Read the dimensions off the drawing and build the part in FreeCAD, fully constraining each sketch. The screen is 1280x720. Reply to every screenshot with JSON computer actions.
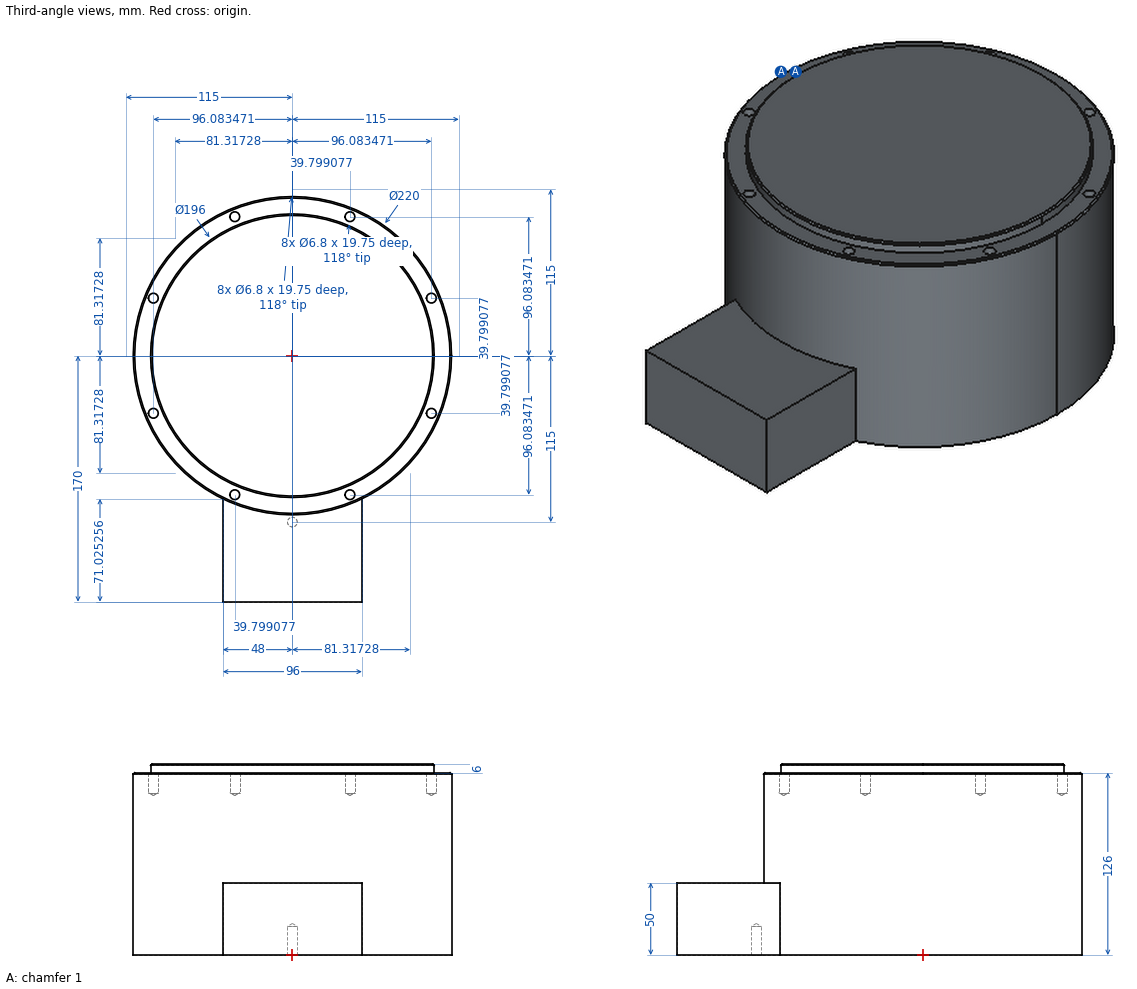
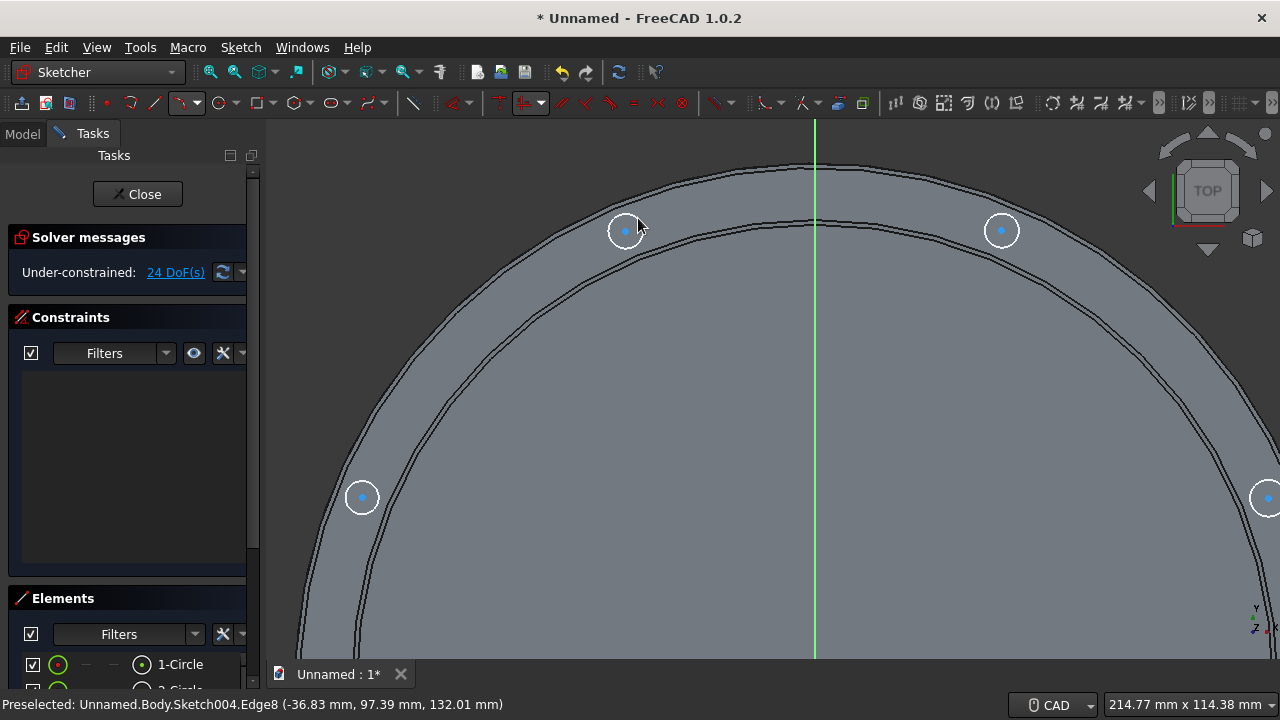
{"action": "left_click", "coordinate": [1014, 219]}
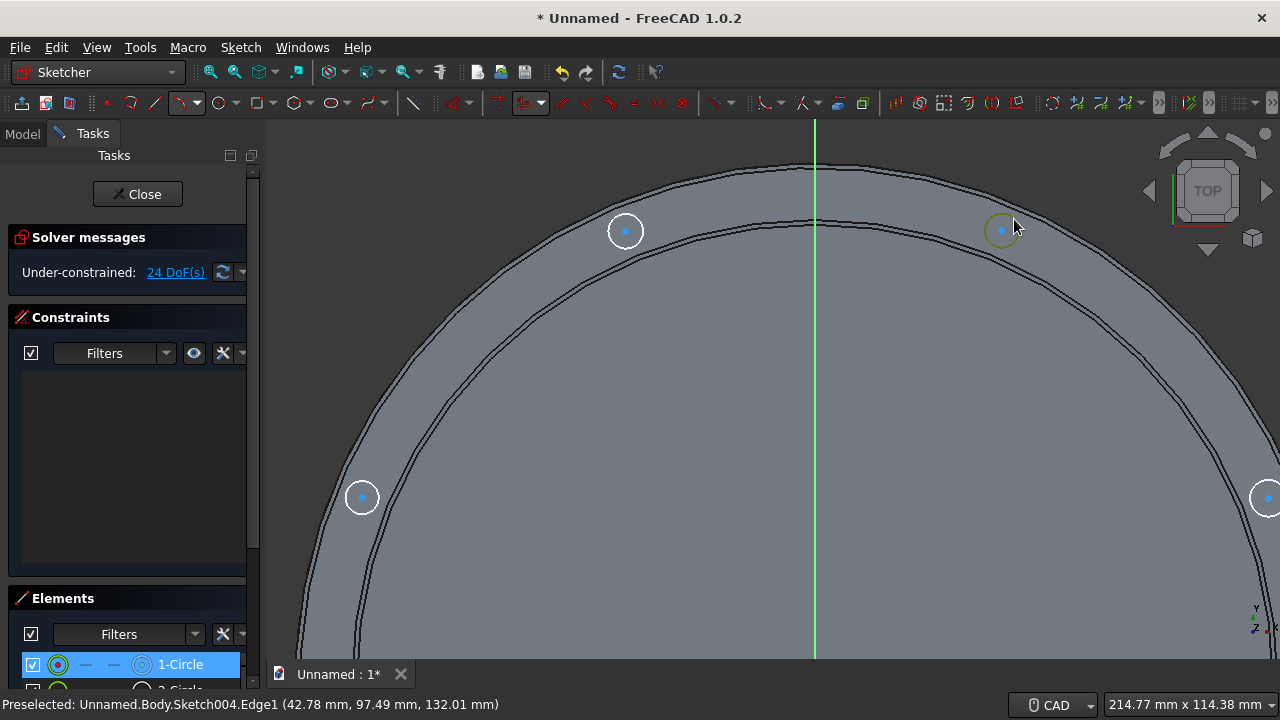
{"action": "scroll", "coordinate": [640, 218], "scroll_direction": "down", "scroll_amount": 5}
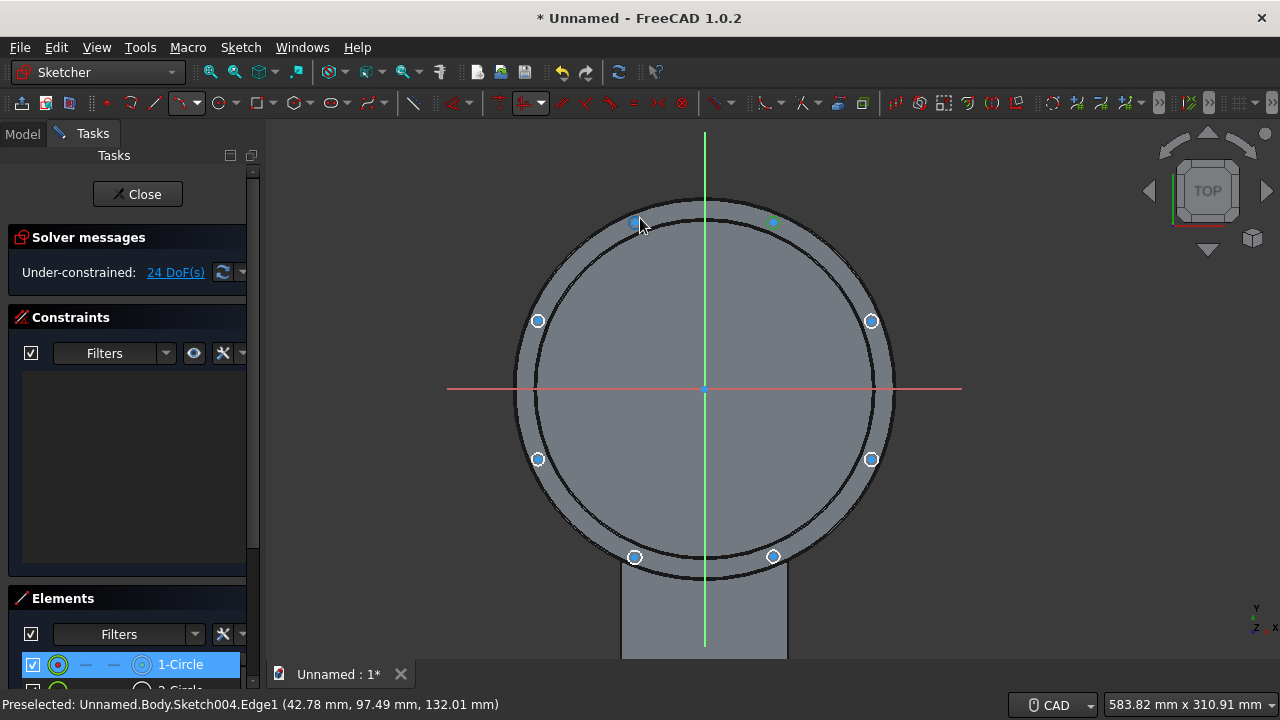
{"action": "scroll", "coordinate": [876, 316], "scroll_direction": "up", "scroll_amount": 4}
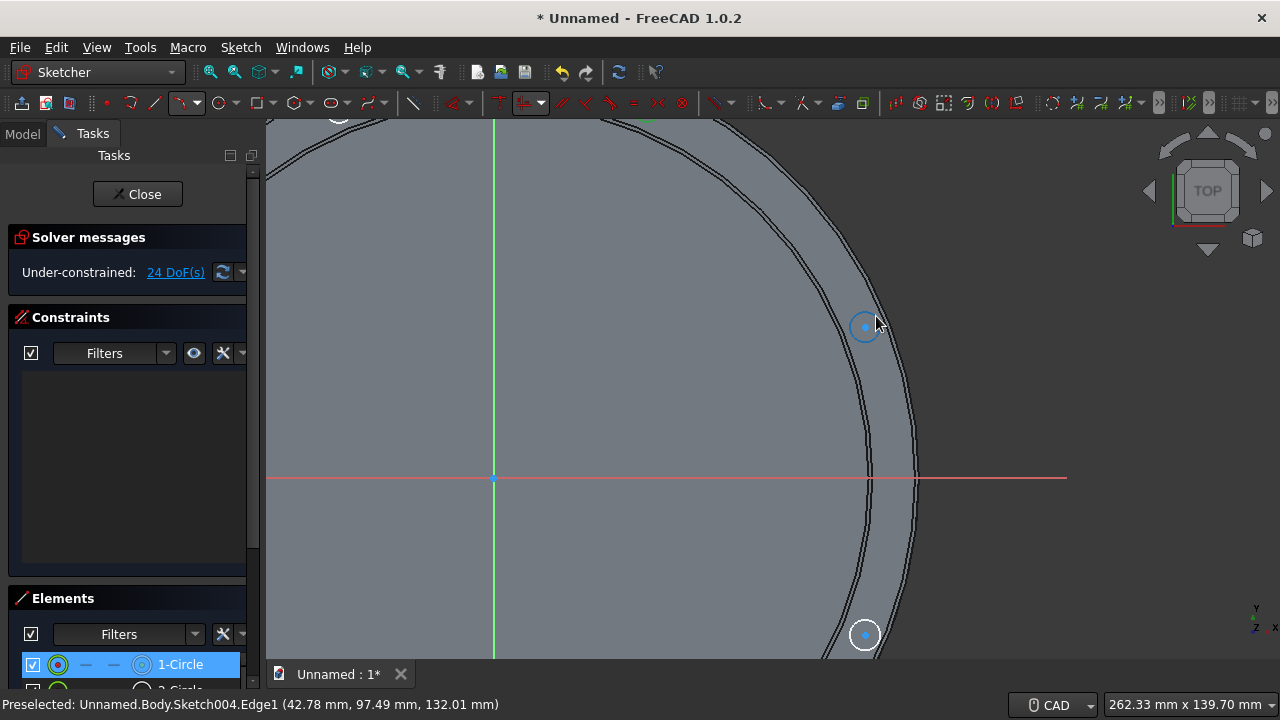
{"action": "left_click", "coordinate": [876, 316]}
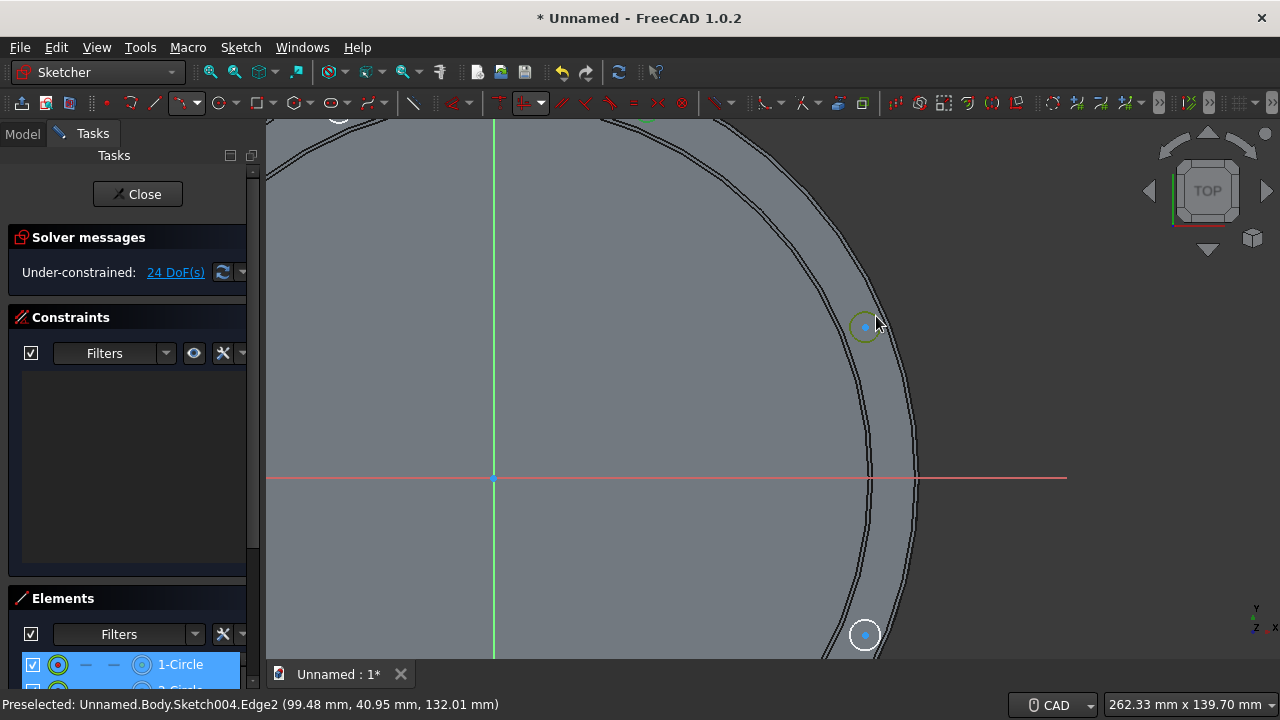
{"action": "left_click", "coordinate": [876, 624]}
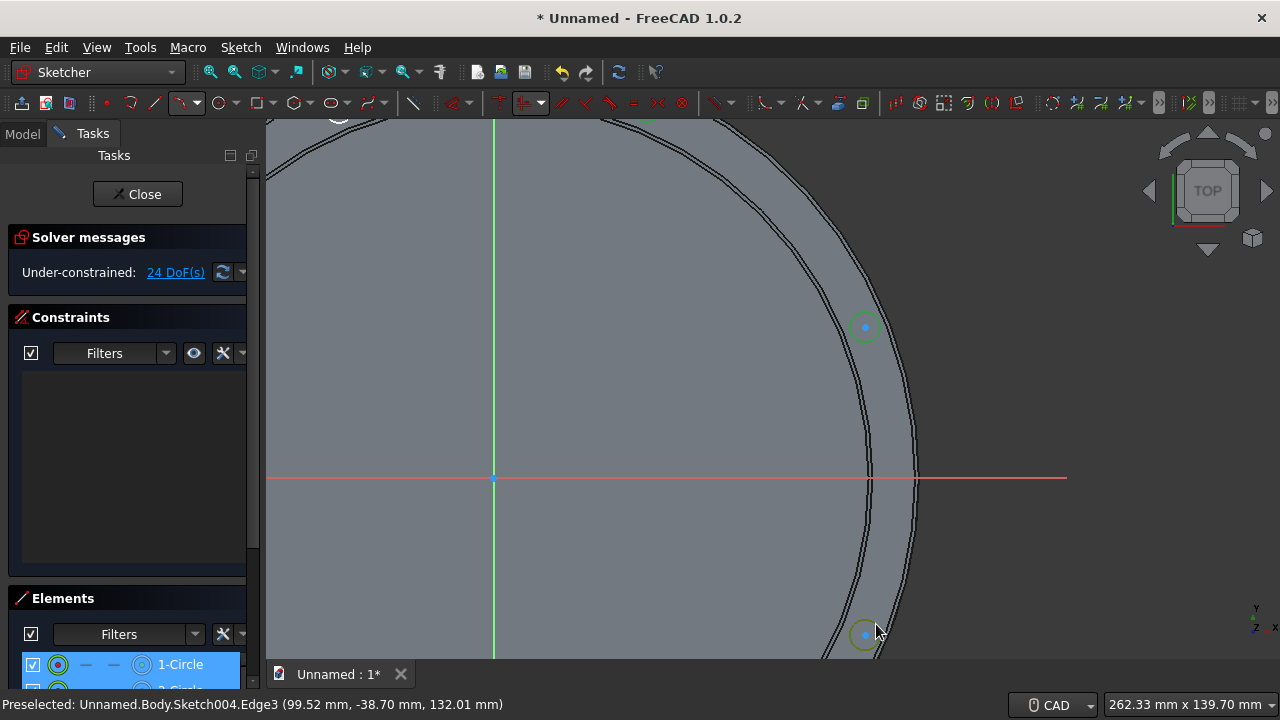
{"action": "scroll", "coordinate": [877, 316], "scroll_direction": "down", "scroll_amount": 4}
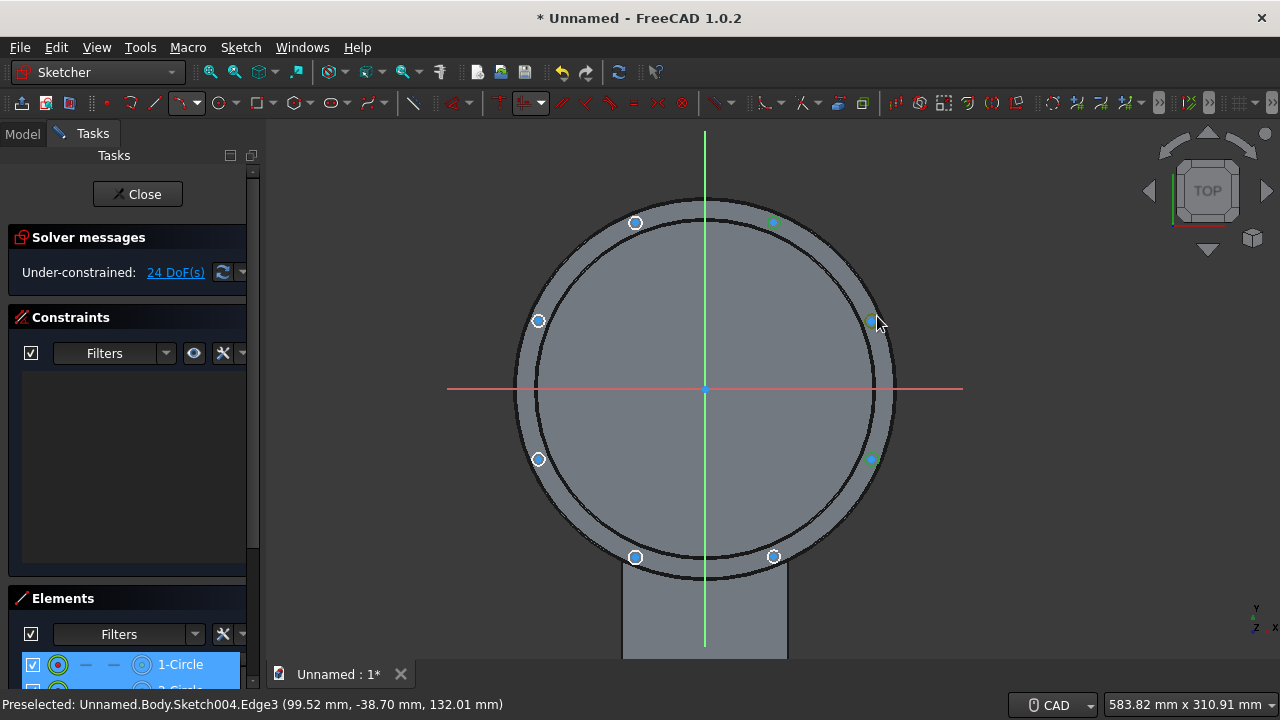
{"action": "scroll", "coordinate": [778, 552], "scroll_direction": "up", "scroll_amount": 4}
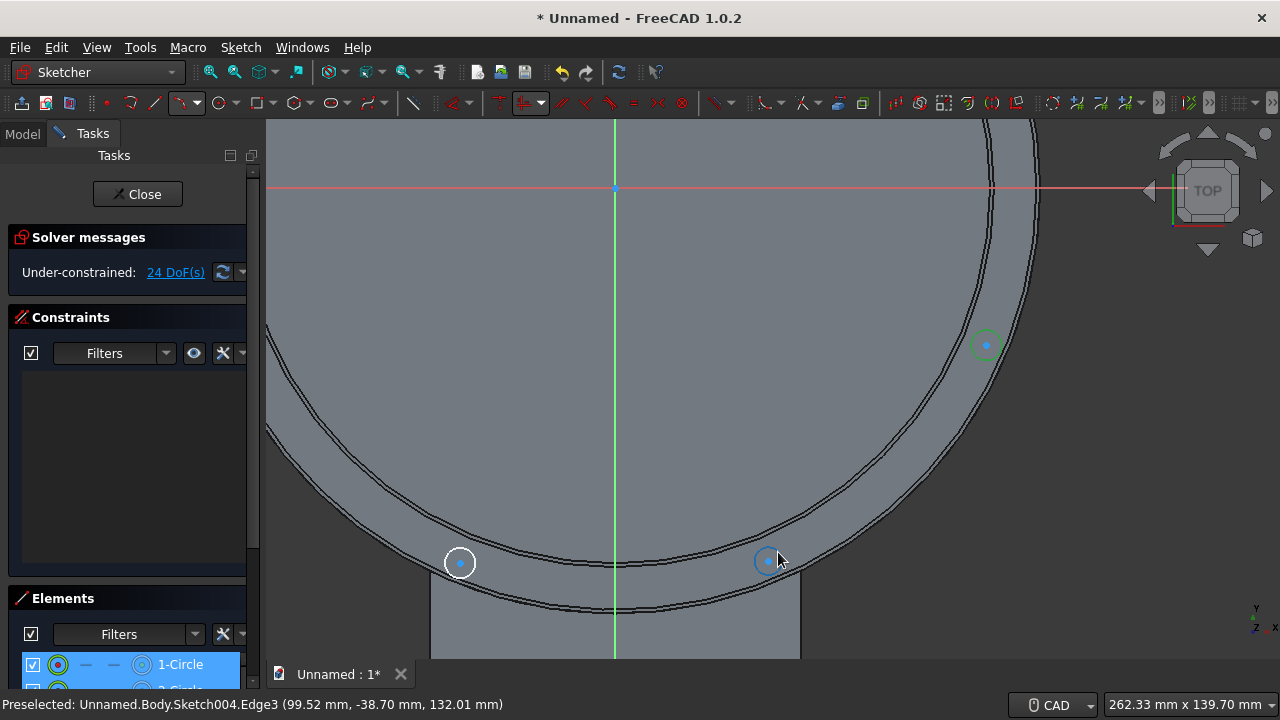
{"action": "left_click", "coordinate": [778, 551]}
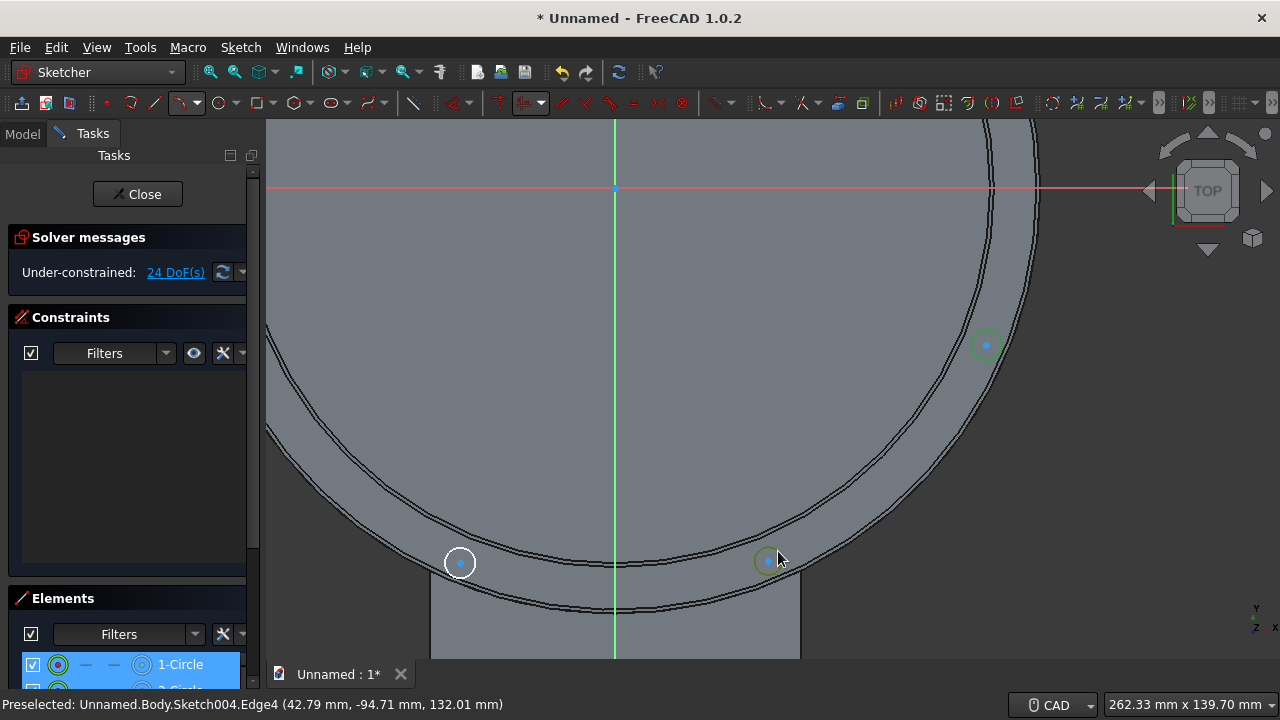
{"action": "left_click", "coordinate": [471, 552]}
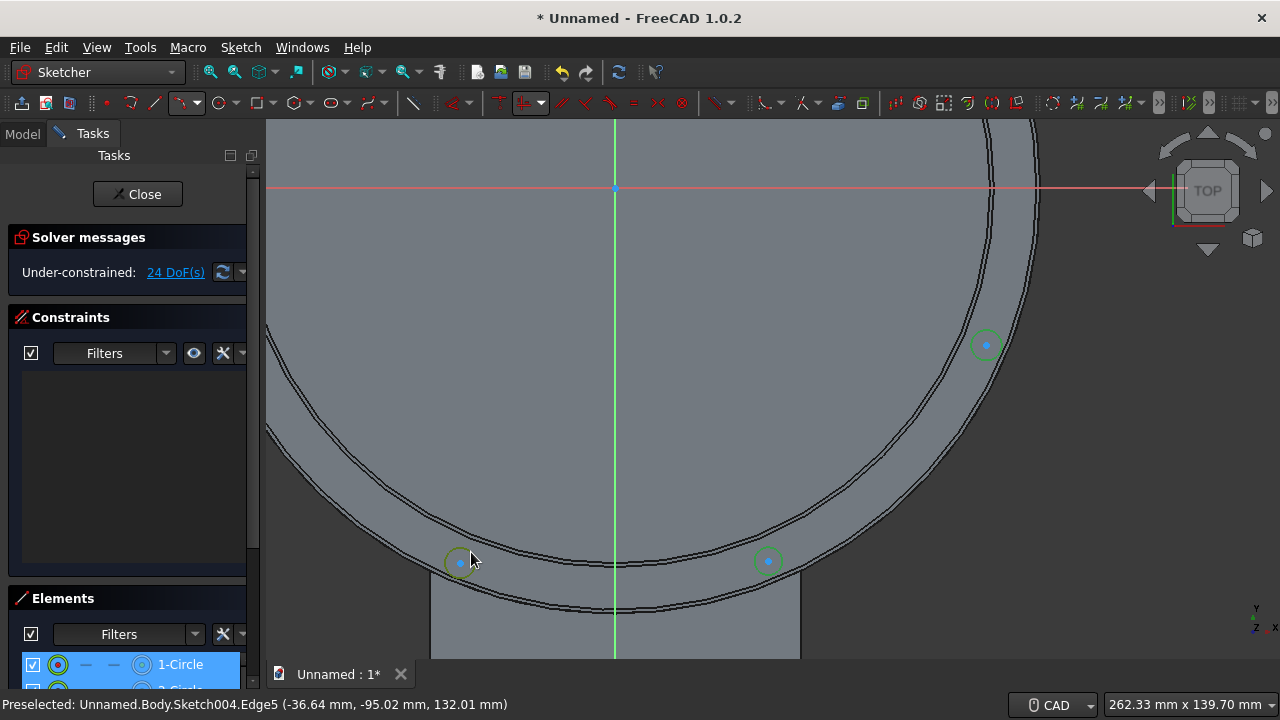
{"action": "scroll", "coordinate": [777, 553], "scroll_direction": "down", "scroll_amount": 4}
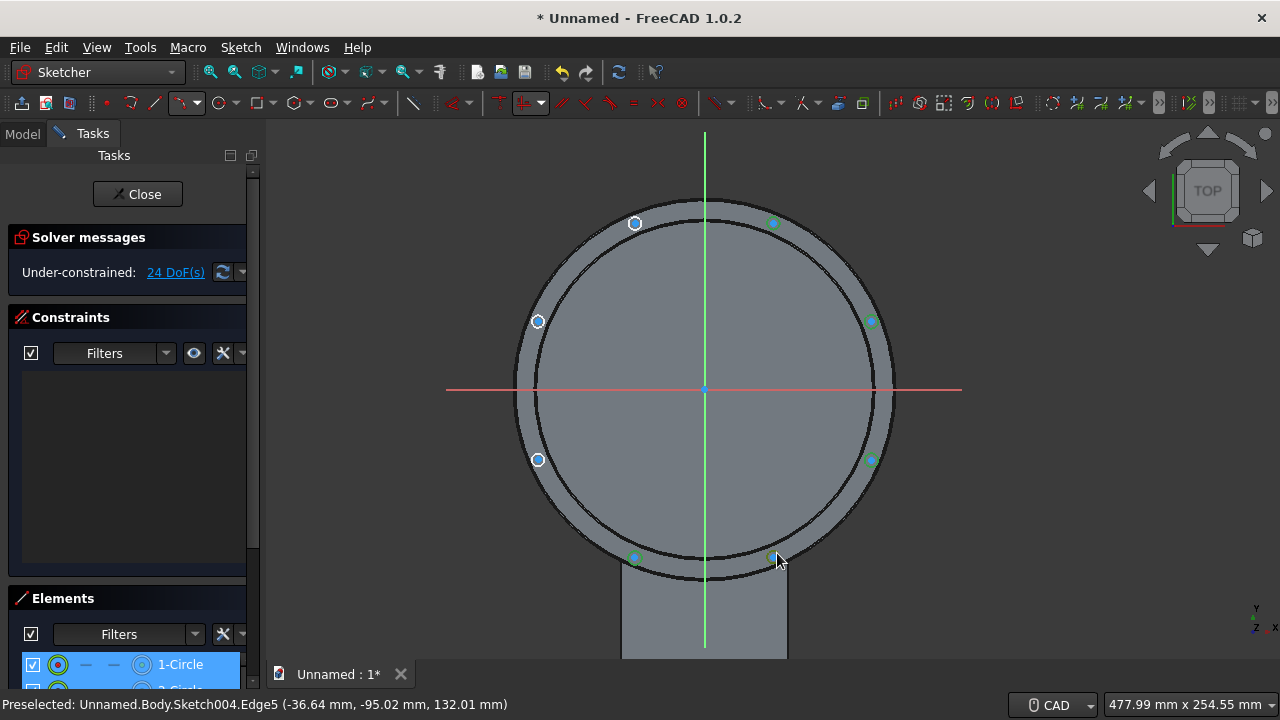
{"action": "scroll", "coordinate": [542, 455], "scroll_direction": "up", "scroll_amount": 4}